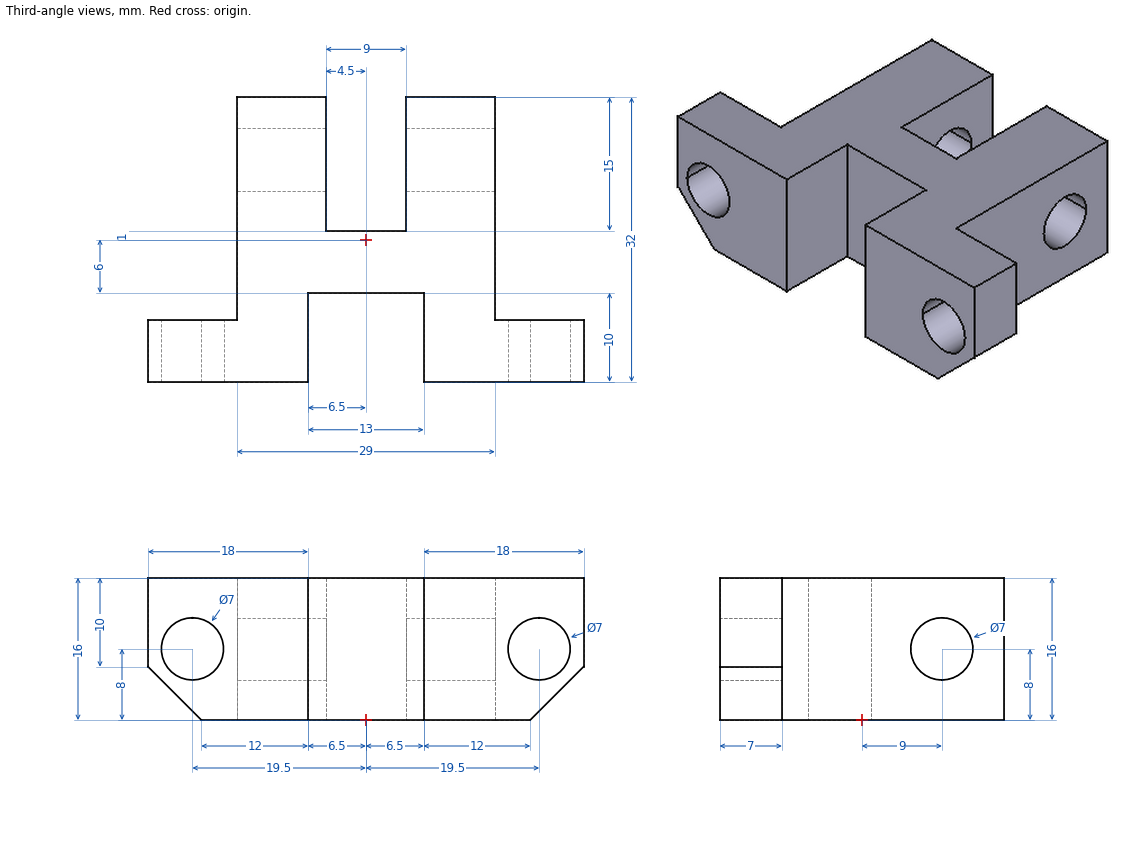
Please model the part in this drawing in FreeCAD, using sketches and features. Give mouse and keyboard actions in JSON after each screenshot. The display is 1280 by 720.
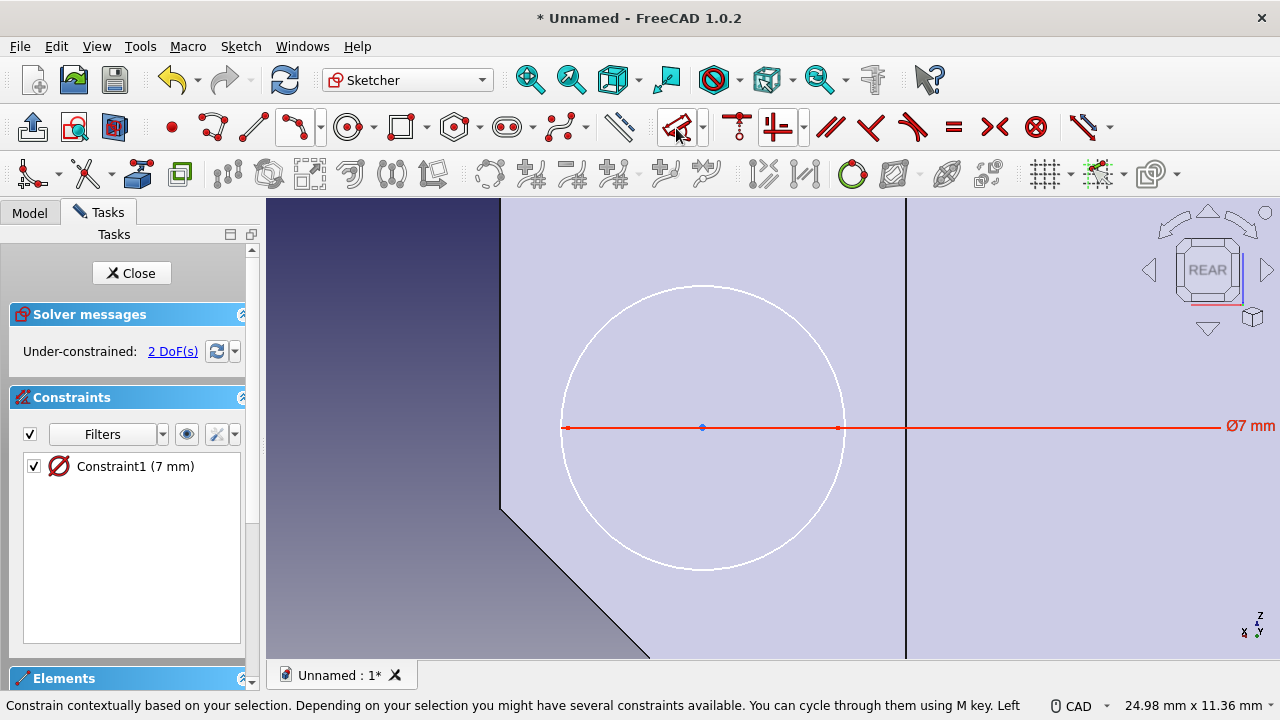
{"action": "left_click", "coordinate": [703, 428]}
{"action": "left_click", "coordinate": [669, 529]}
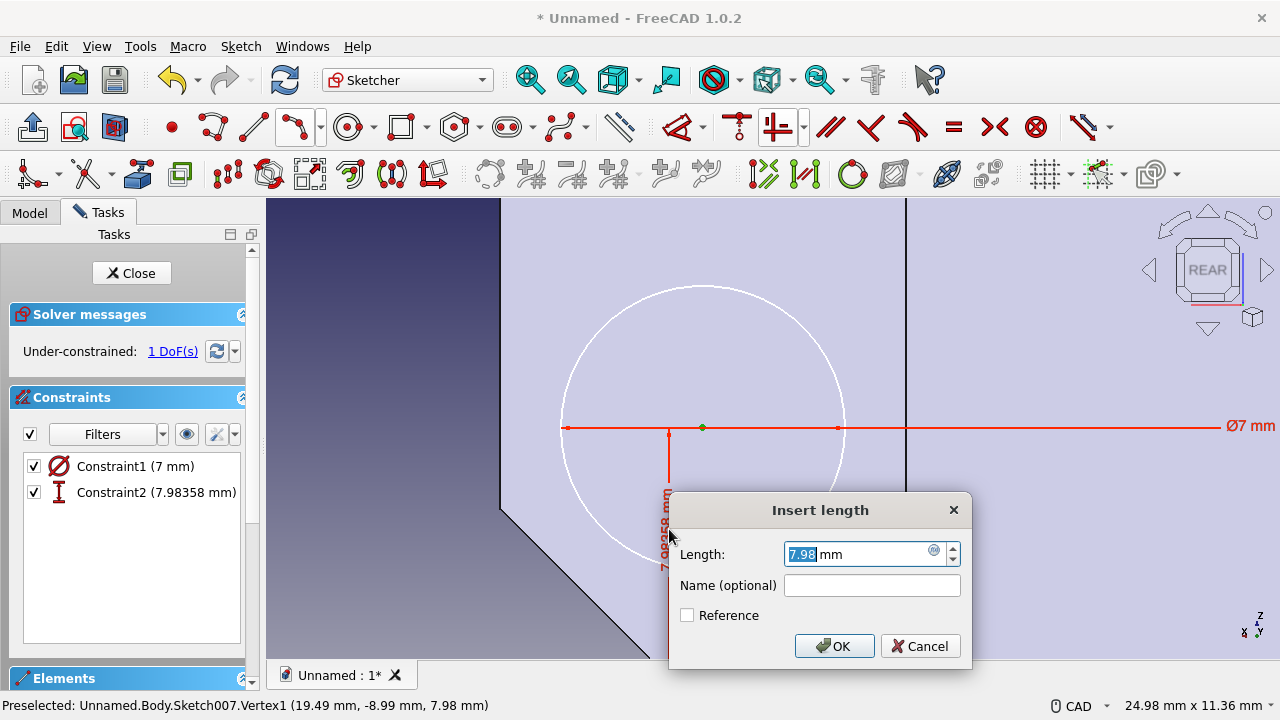
{"action": "type", "text": "8"}
{"action": "key", "text": "Return"}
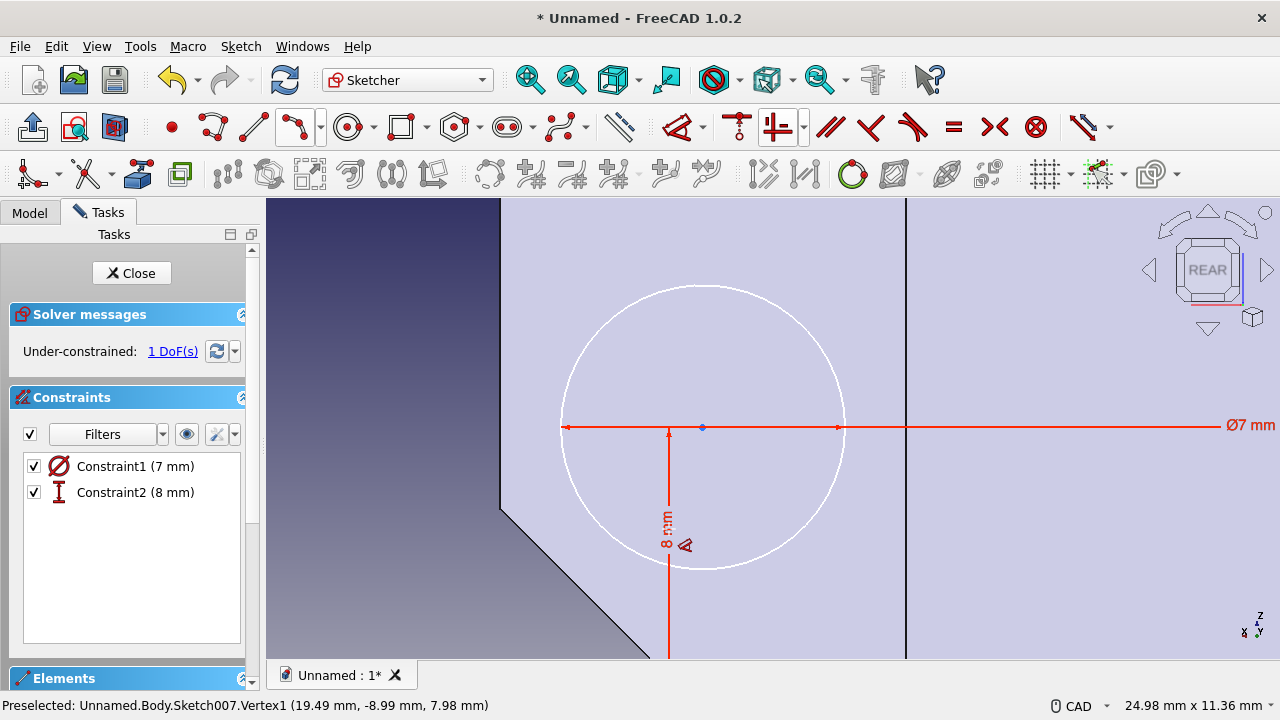
{"action": "left_click", "coordinate": [703, 427]}
{"action": "left_click", "coordinate": [909, 393]}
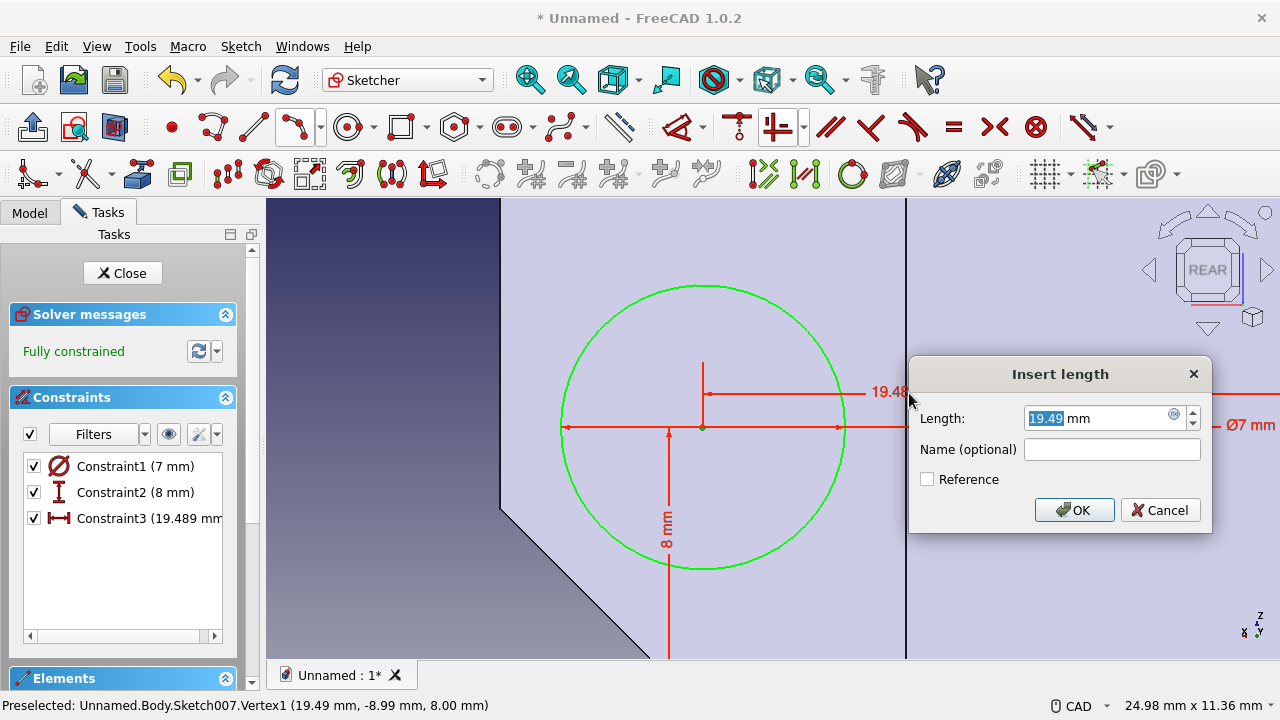
{"action": "type", "text": "19.5"}
{"action": "key", "text": "Return"}
{"action": "key", "text": "Escape"}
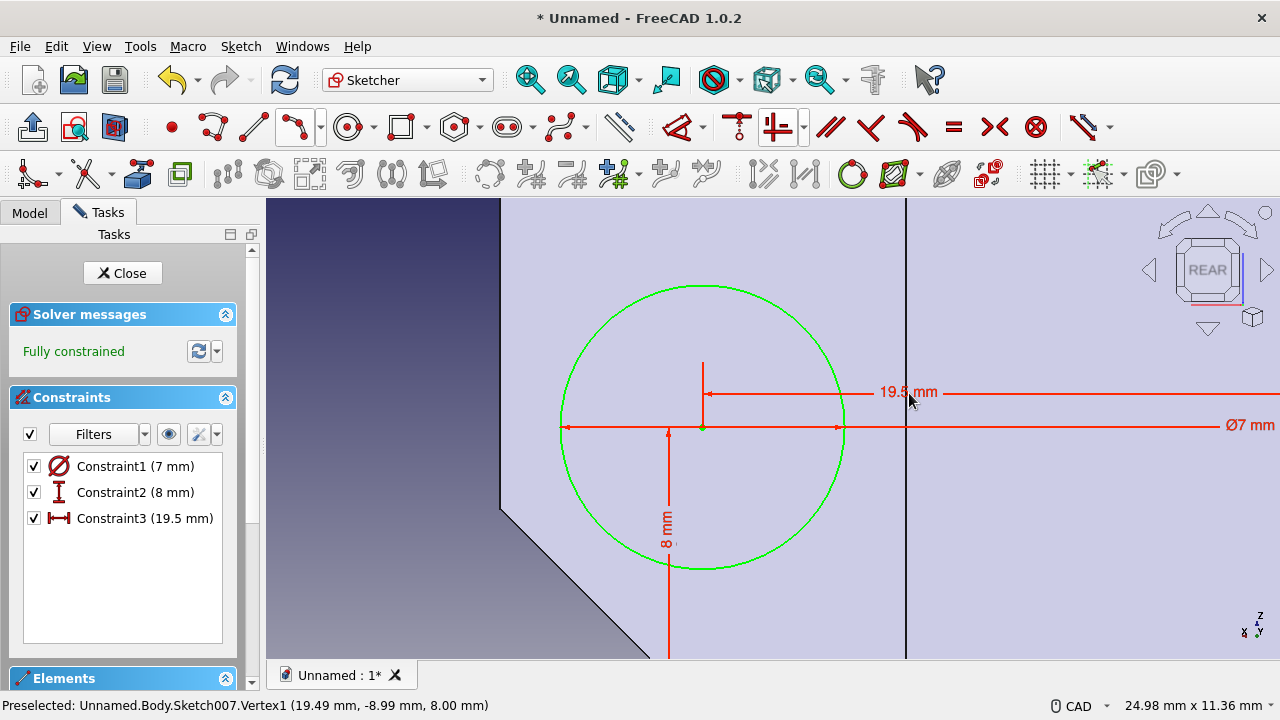
{"action": "left_click", "coordinate": [123, 273]}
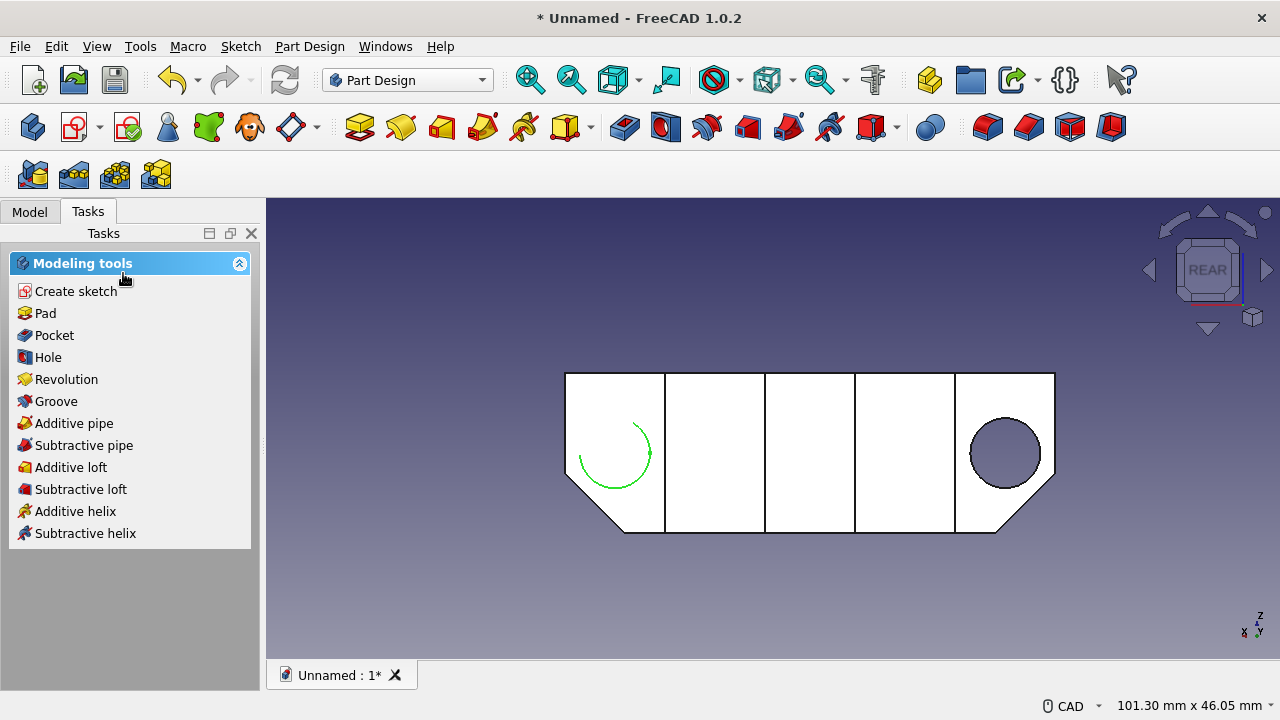
{"action": "left_click", "coordinate": [625, 128]}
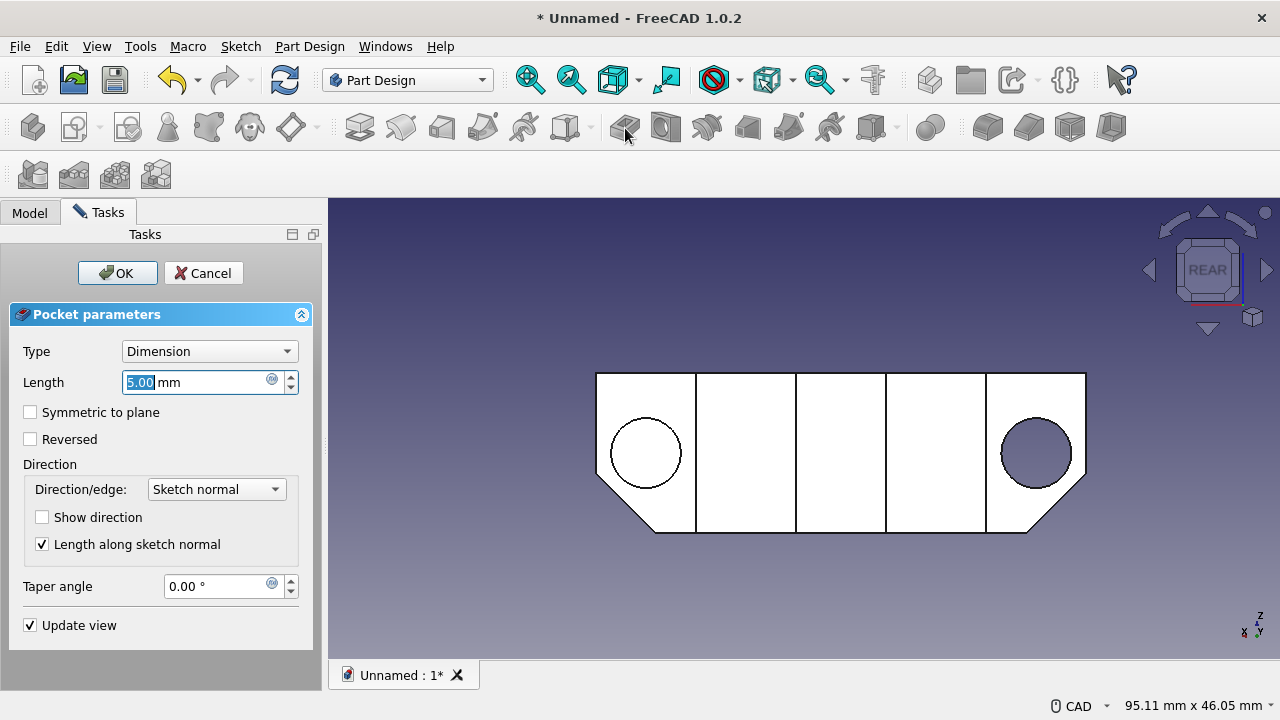
{"action": "type", "text": "7"}
{"action": "key", "text": "Tab"}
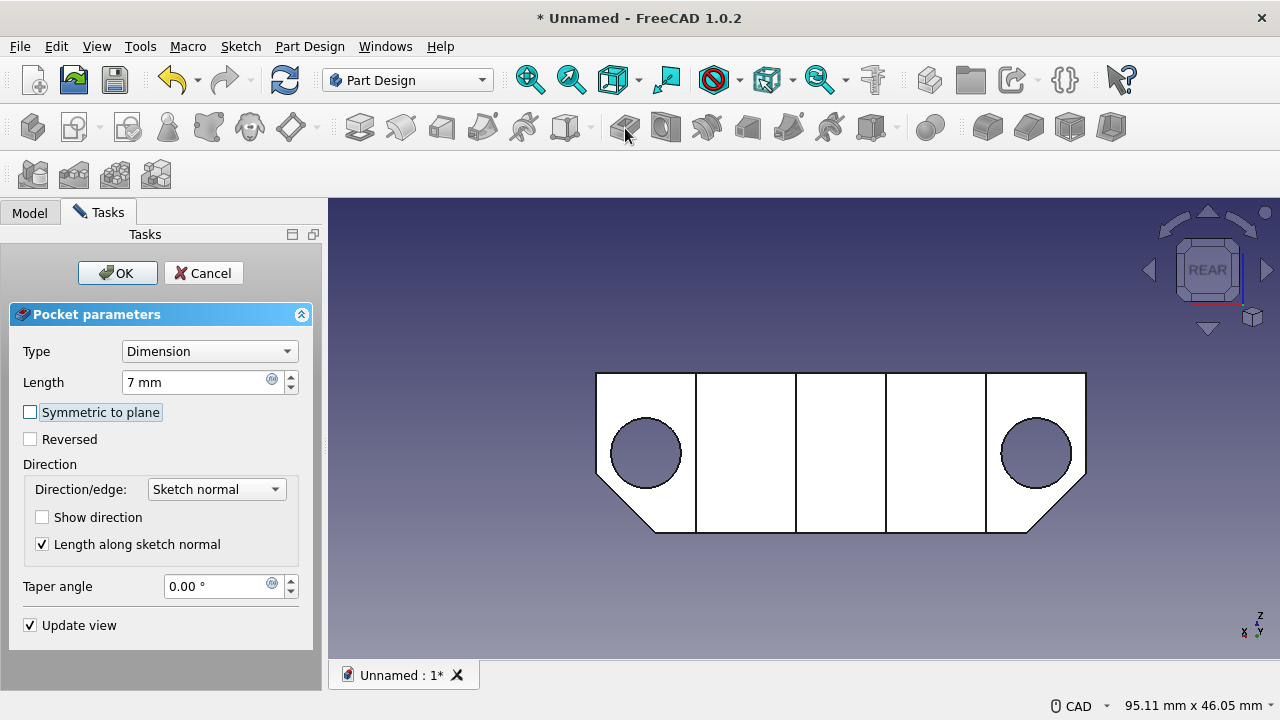
{"action": "left_click", "coordinate": [118, 273]}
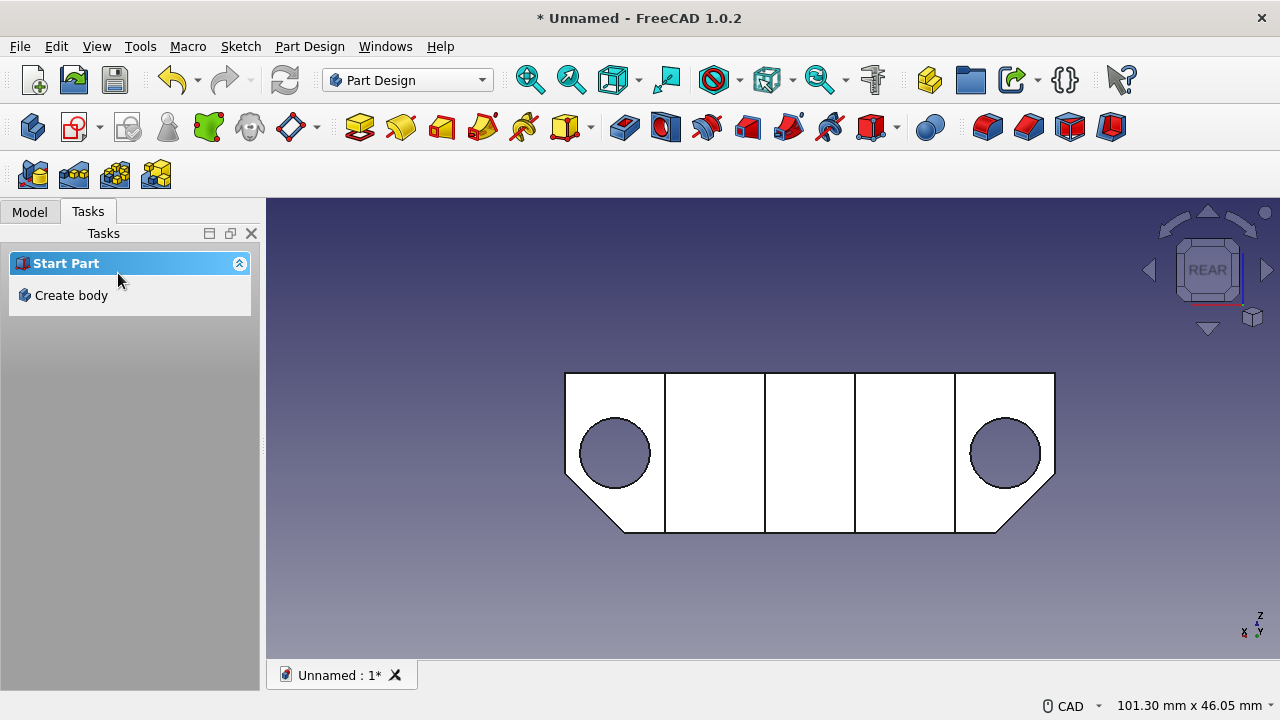
{"action": "key", "text": "0"}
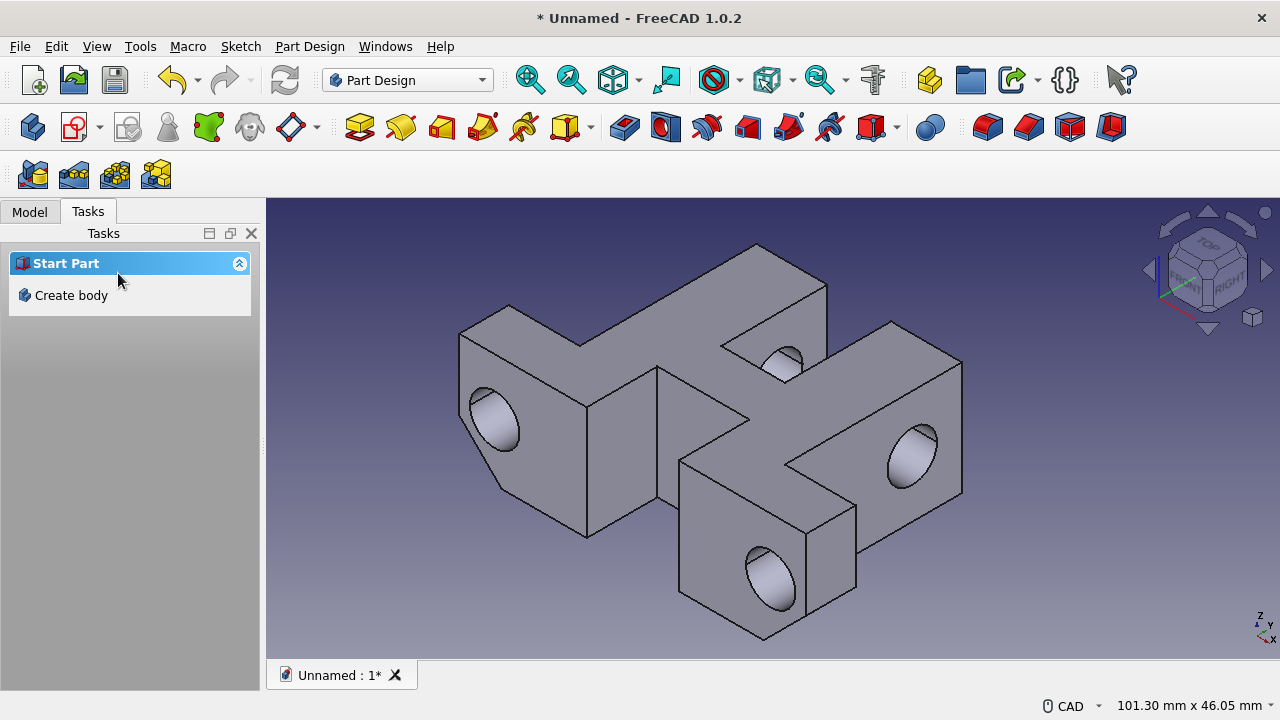
{"action": "left_click", "coordinate": [531, 80]}